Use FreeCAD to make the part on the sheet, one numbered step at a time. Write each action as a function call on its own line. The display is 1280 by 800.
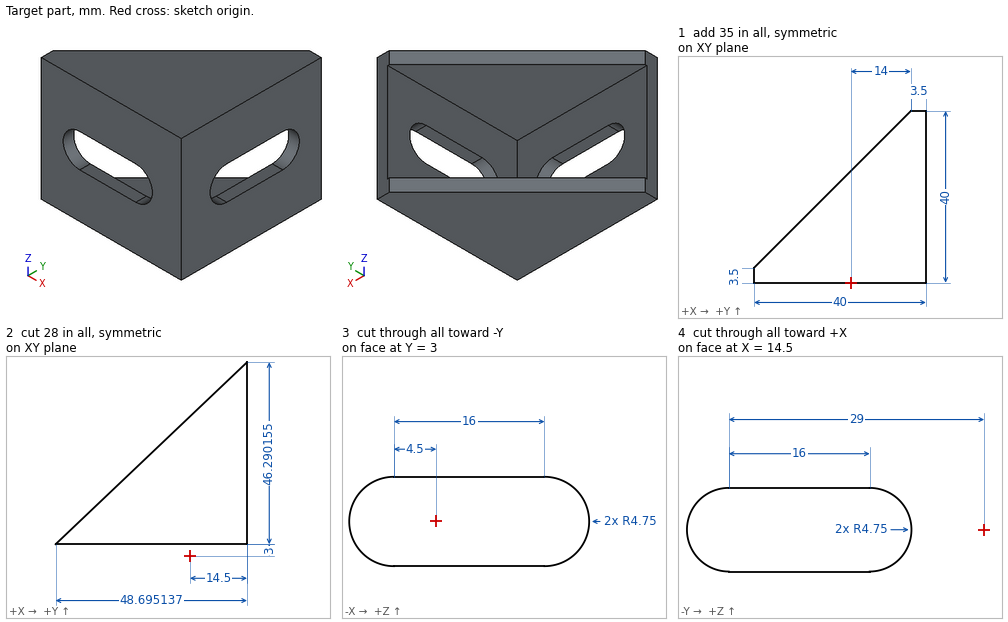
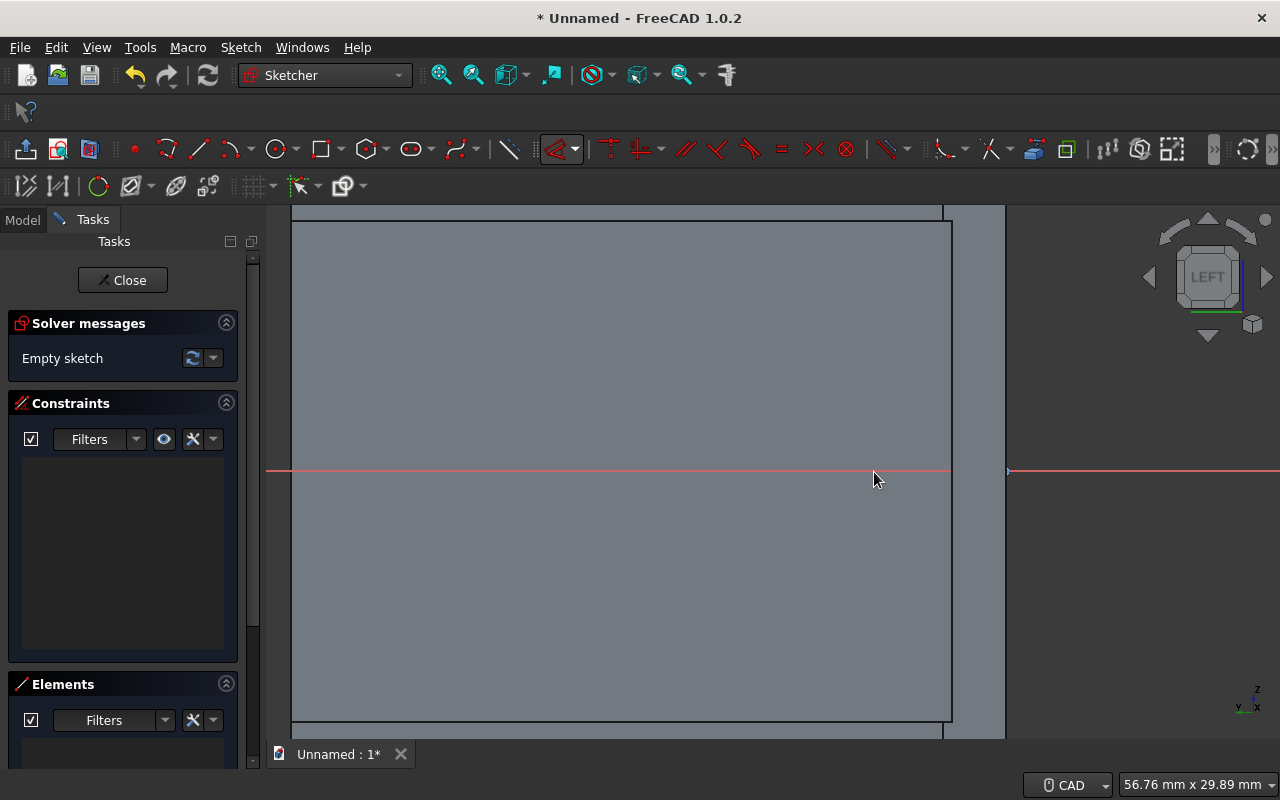
click(488, 471)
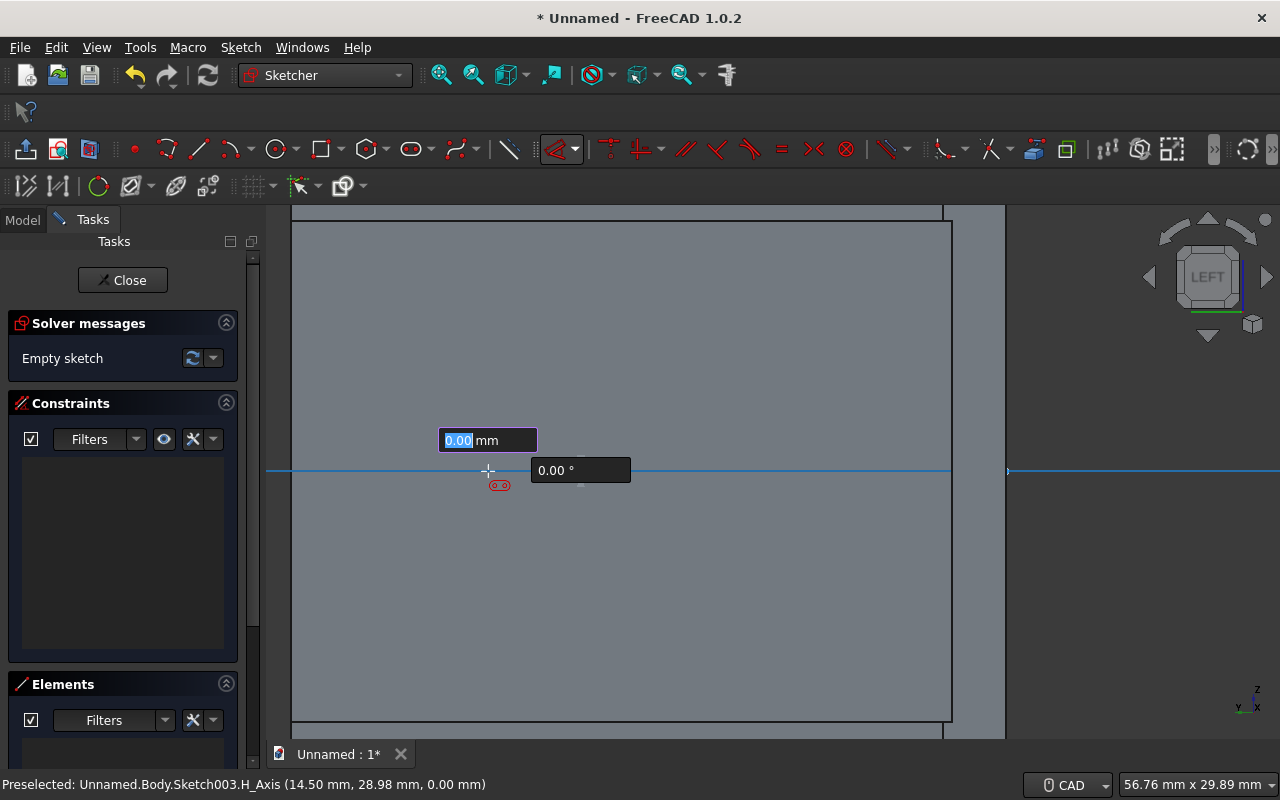
click(774, 462)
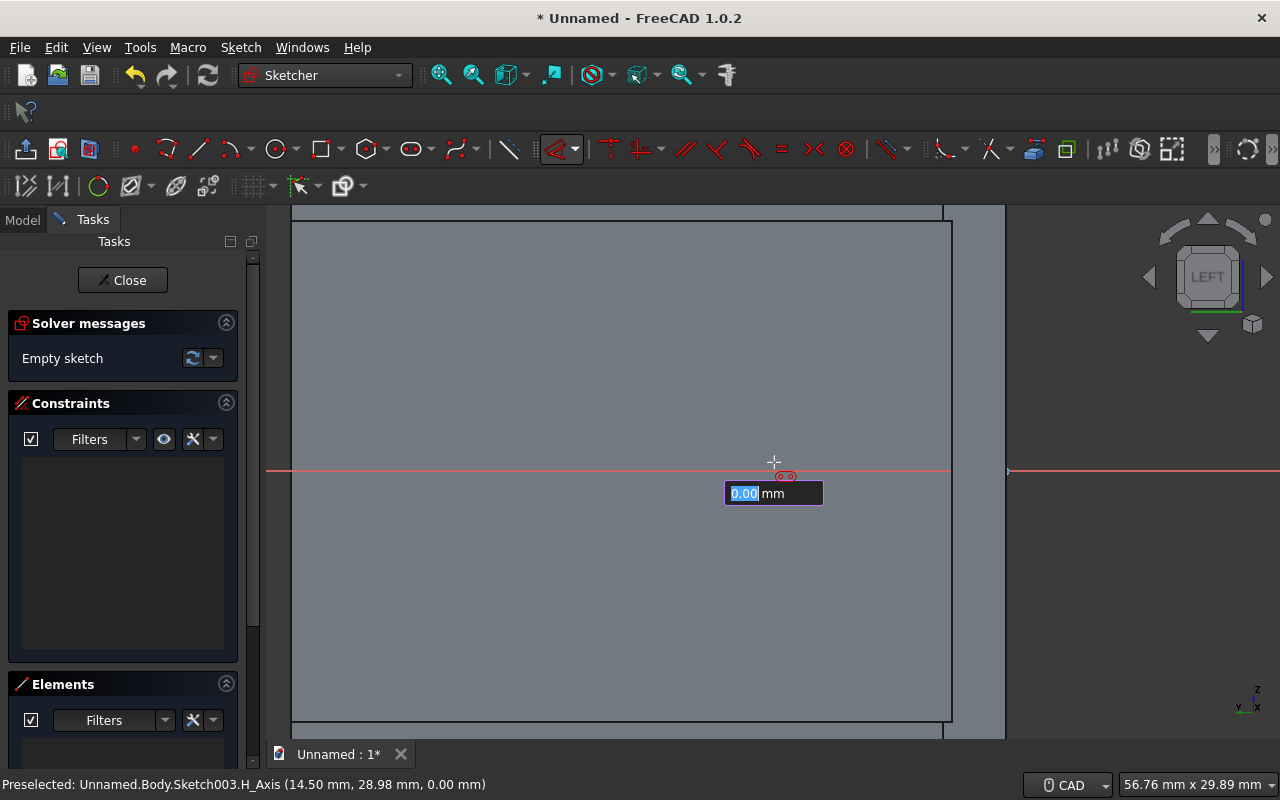
click(631, 556)
key(Escape)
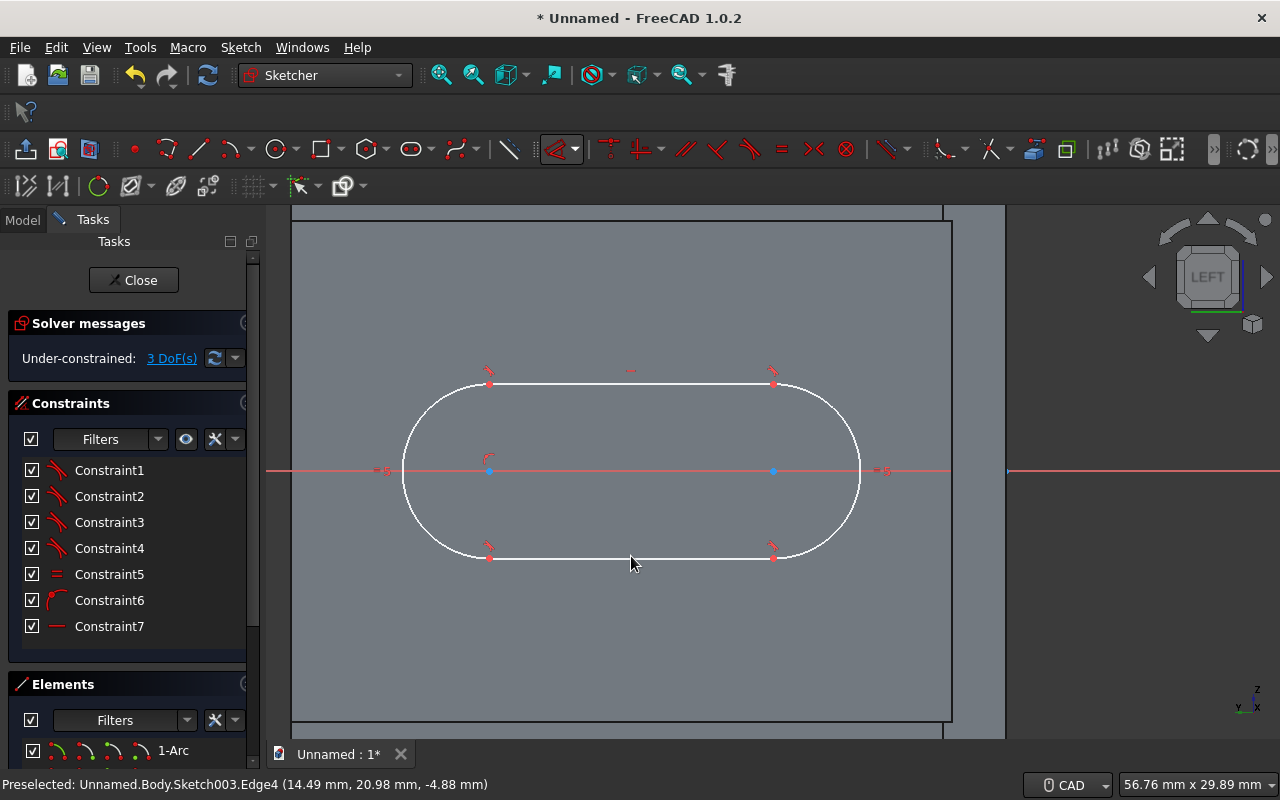
click(419, 420)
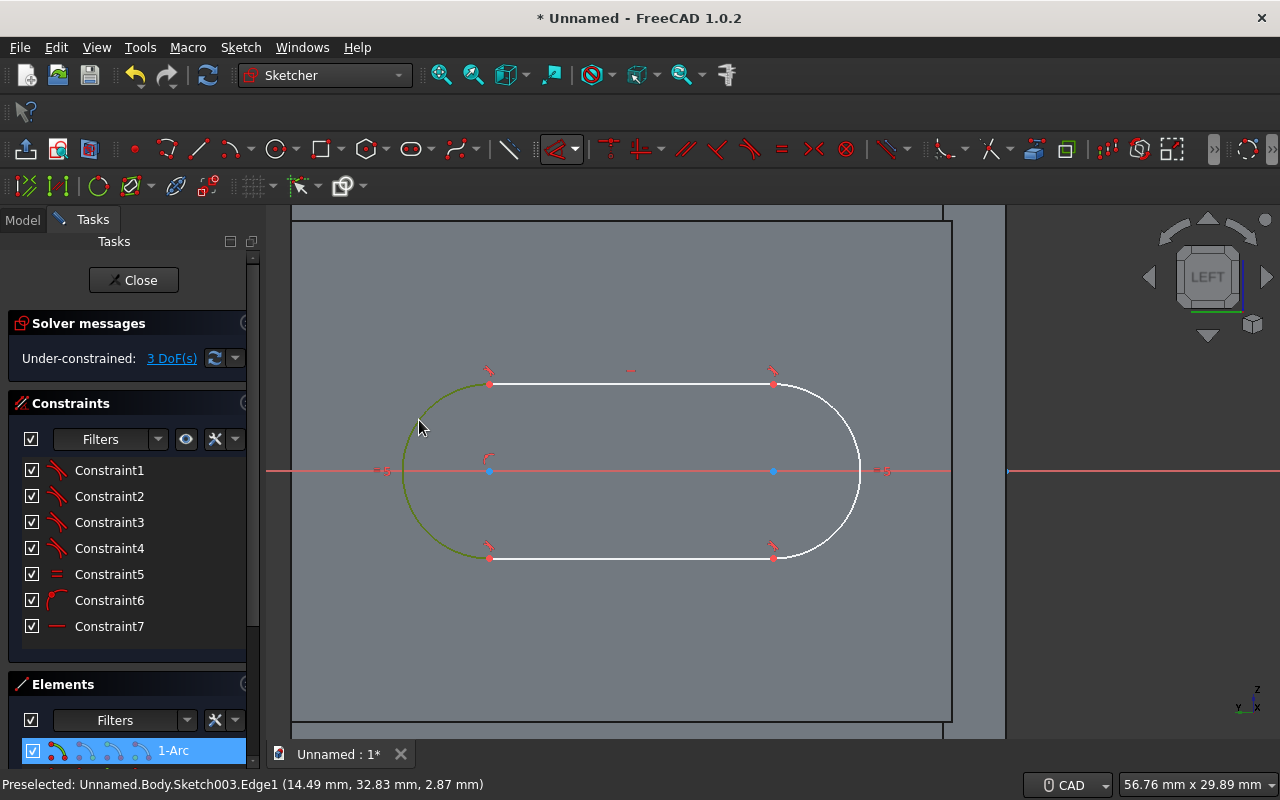
key(k)
key(r)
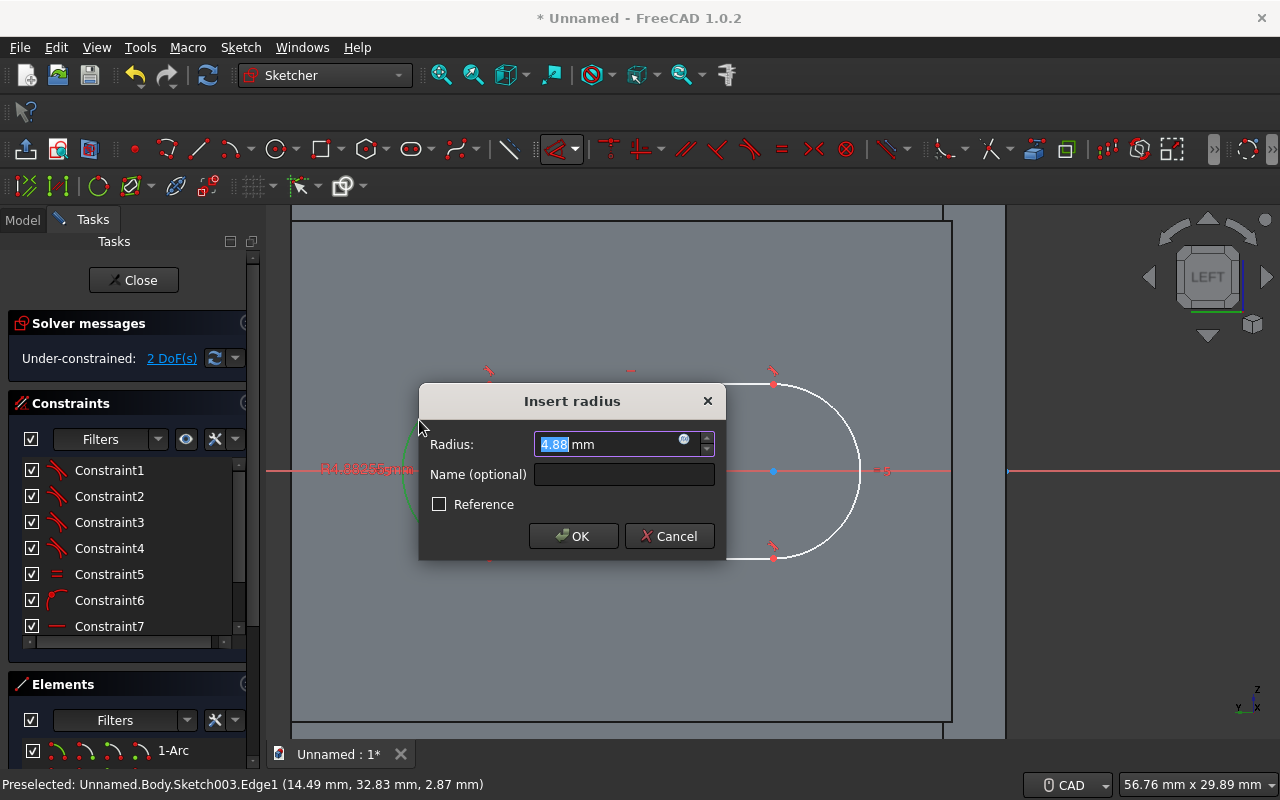
text(4.75)
key(Return)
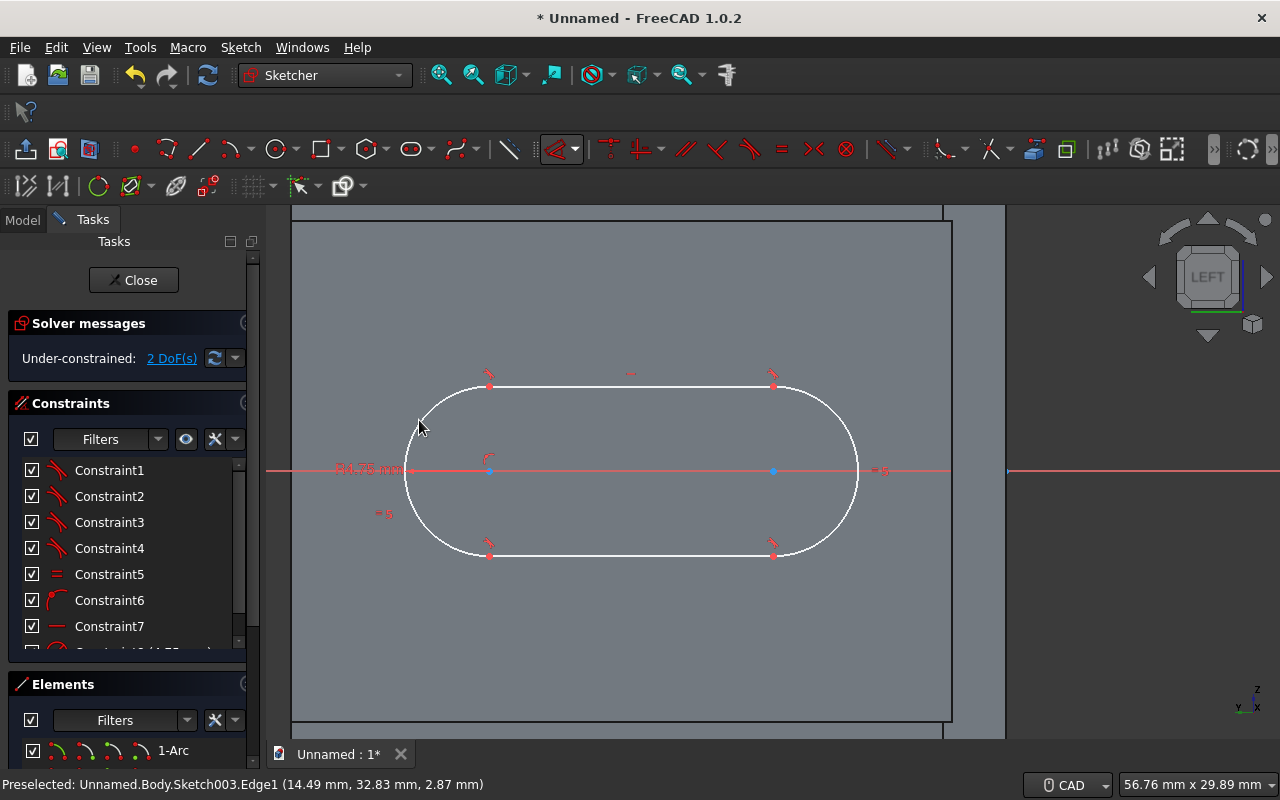
click(575, 387)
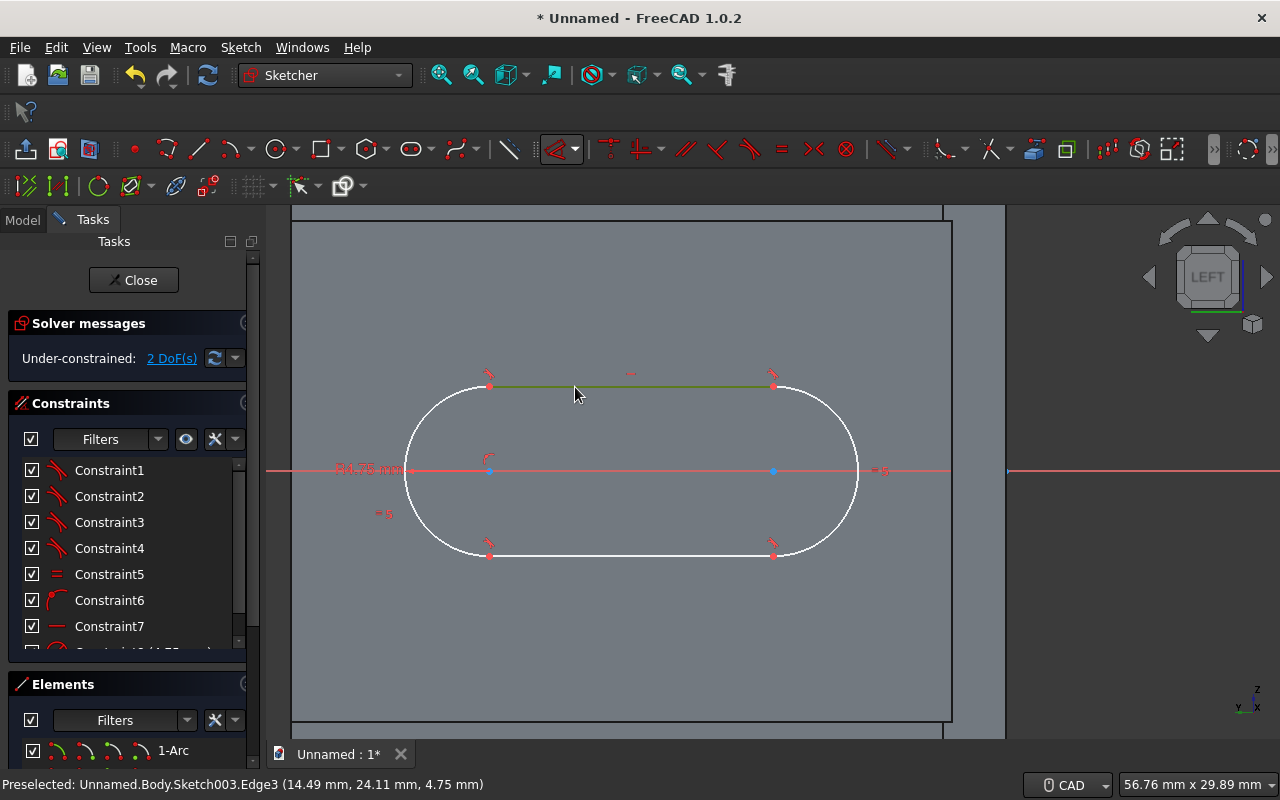
key(l)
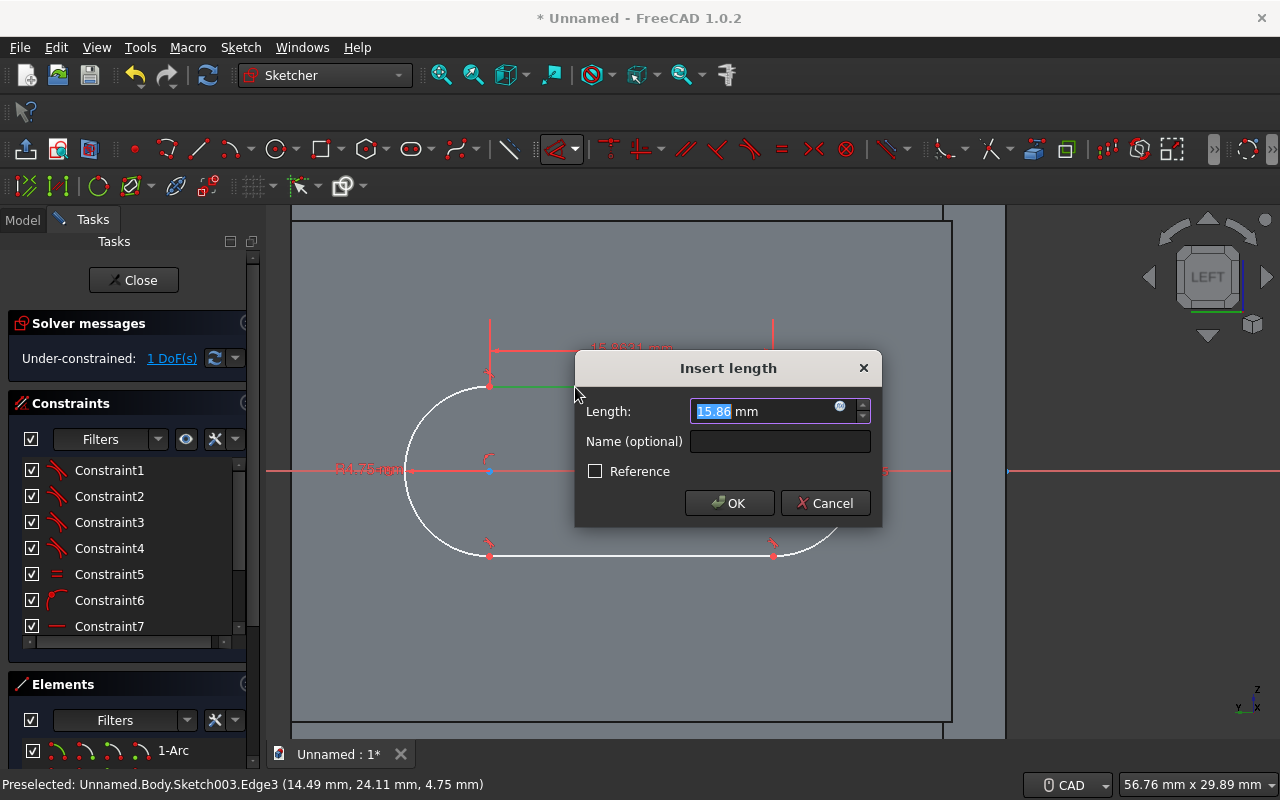
text(16)
key(Return)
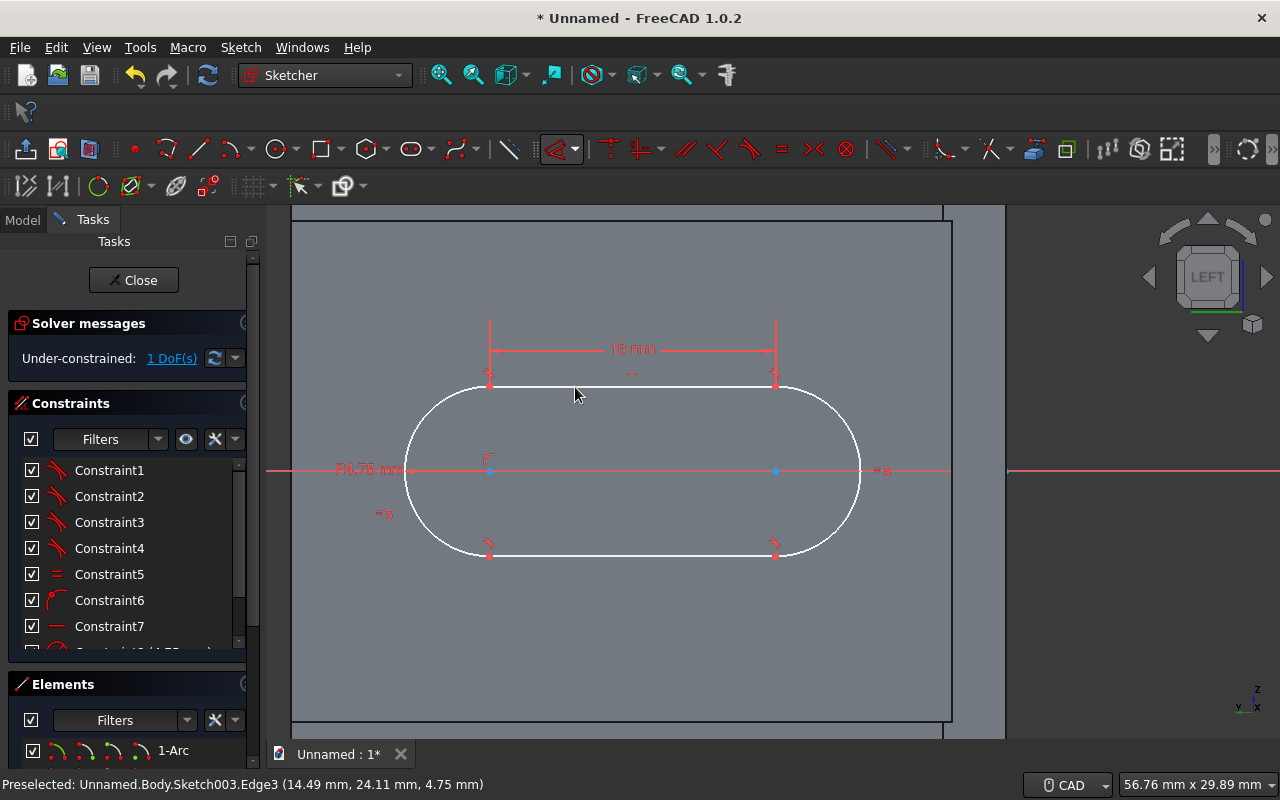
click(490, 387)